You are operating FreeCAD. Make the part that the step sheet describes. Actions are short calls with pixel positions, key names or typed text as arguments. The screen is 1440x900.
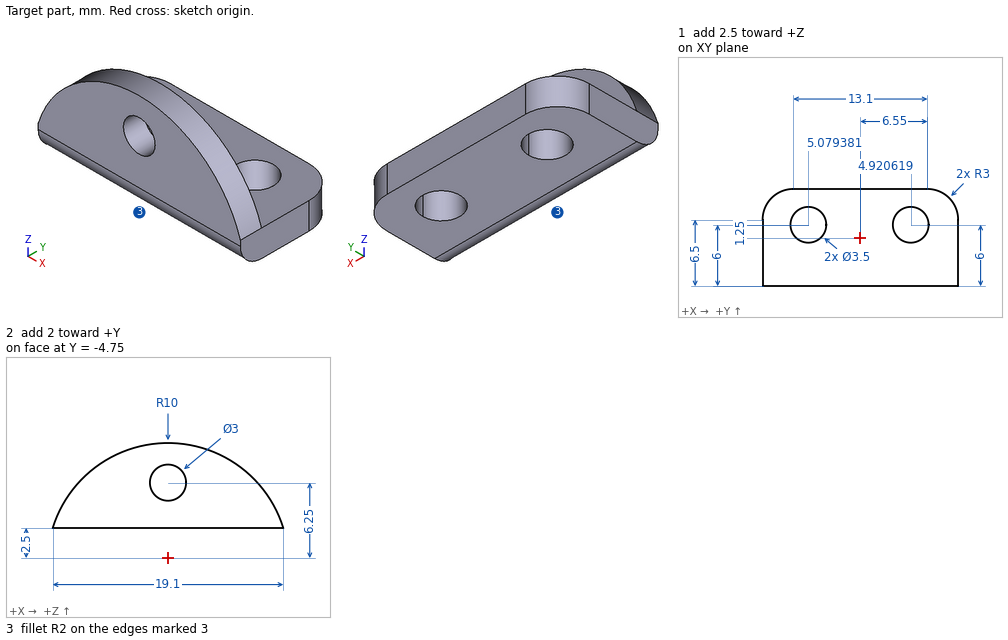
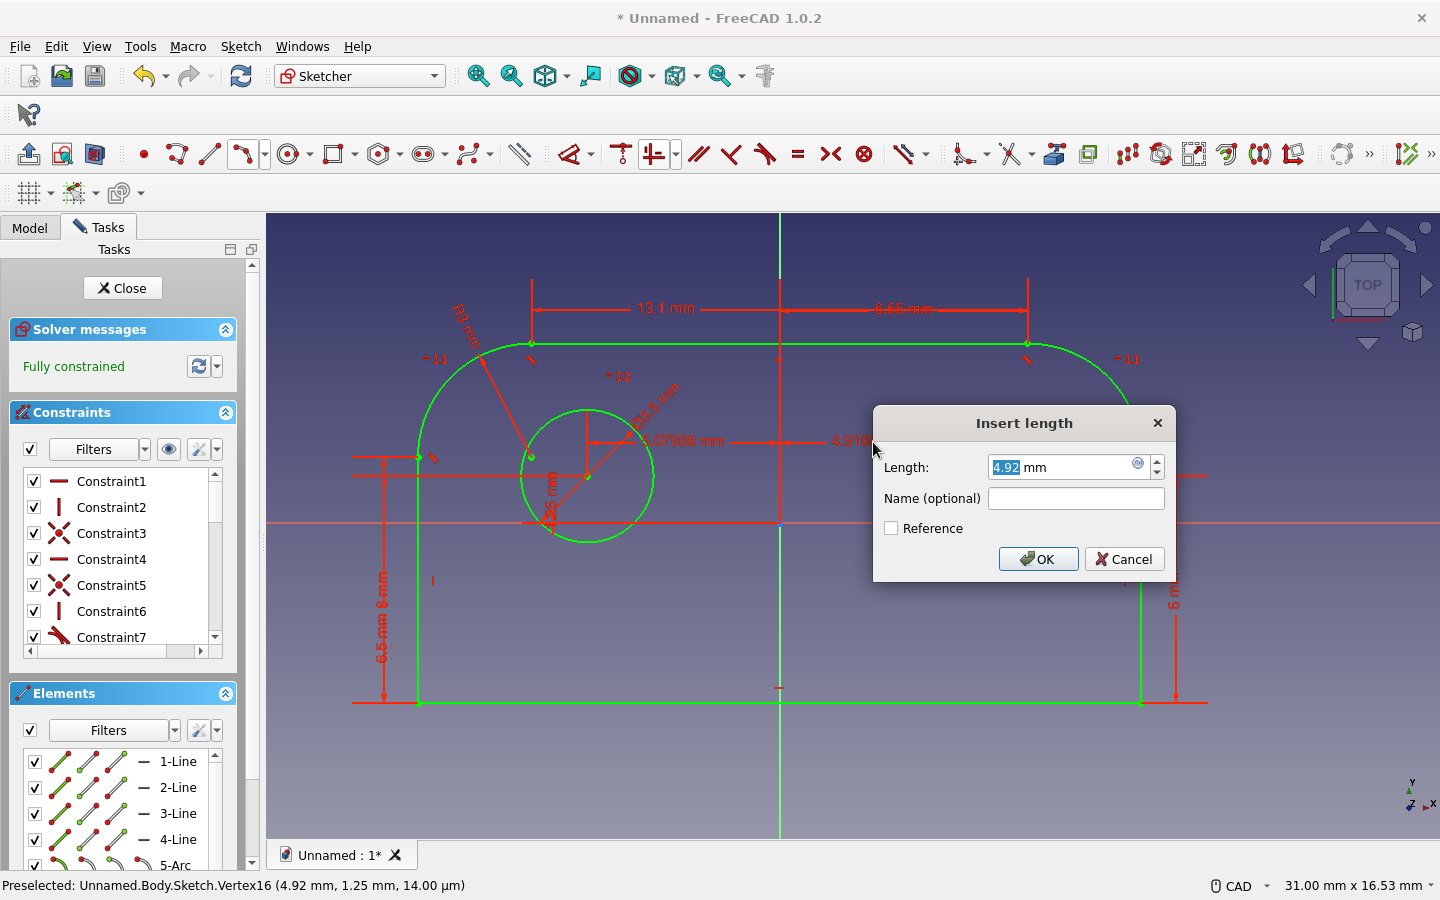
text(4.920619)
key(Return)
key(Escape)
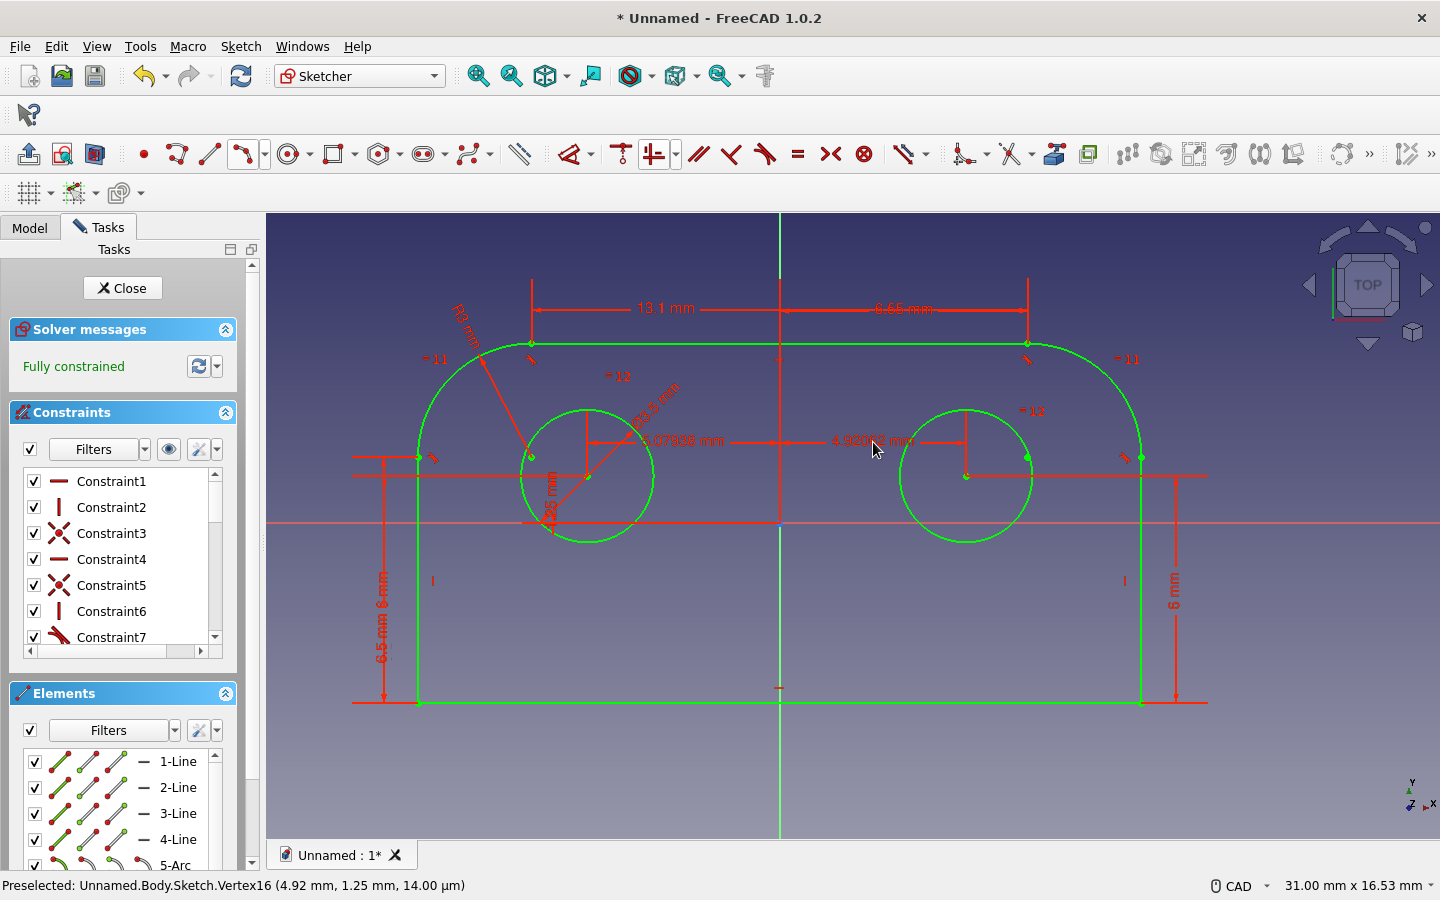
click(123, 288)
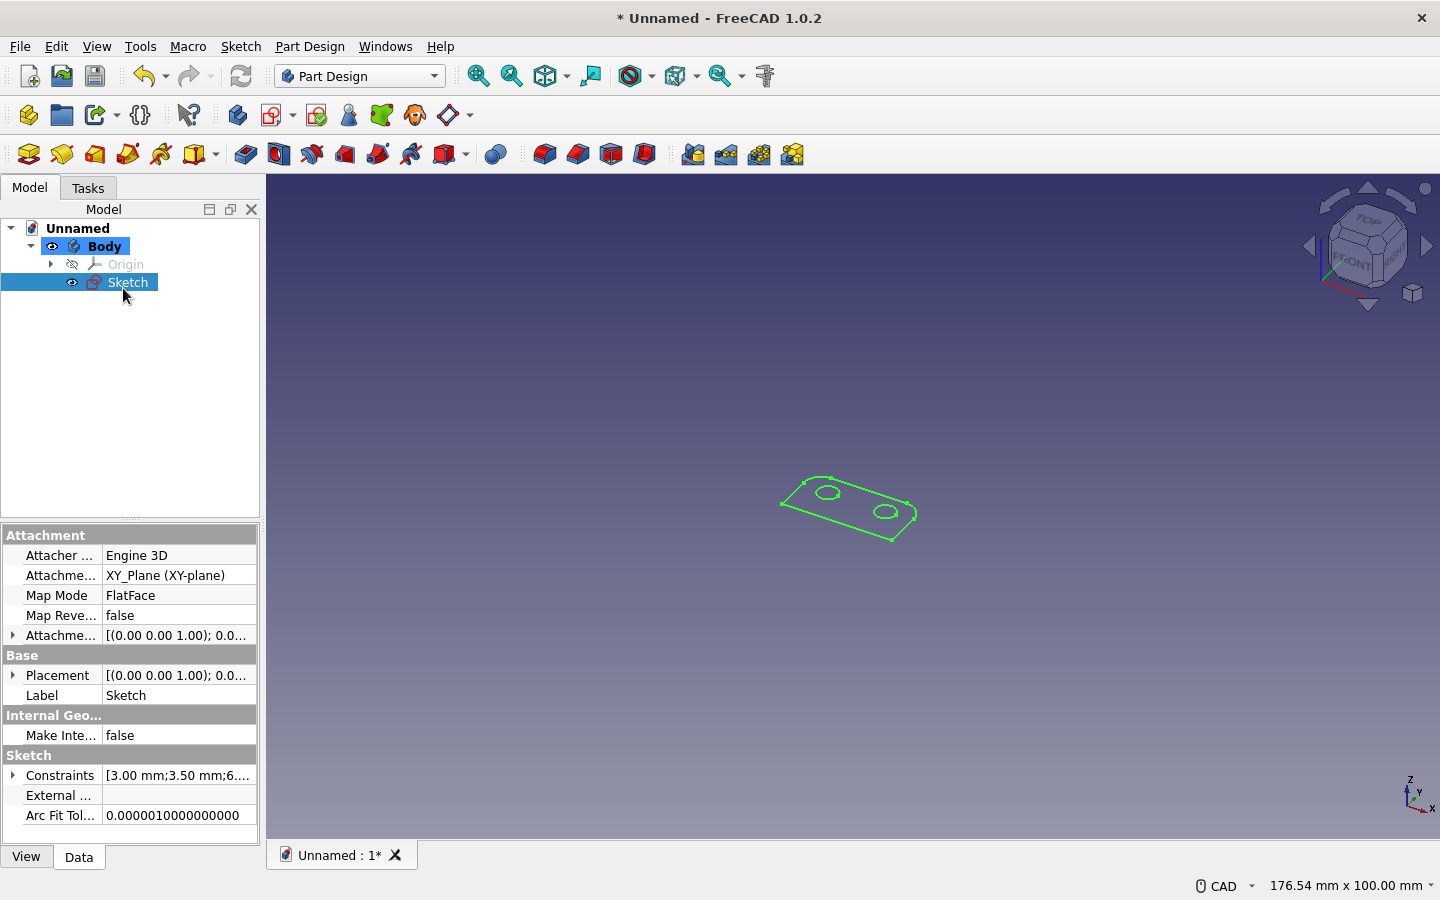
click(29, 154)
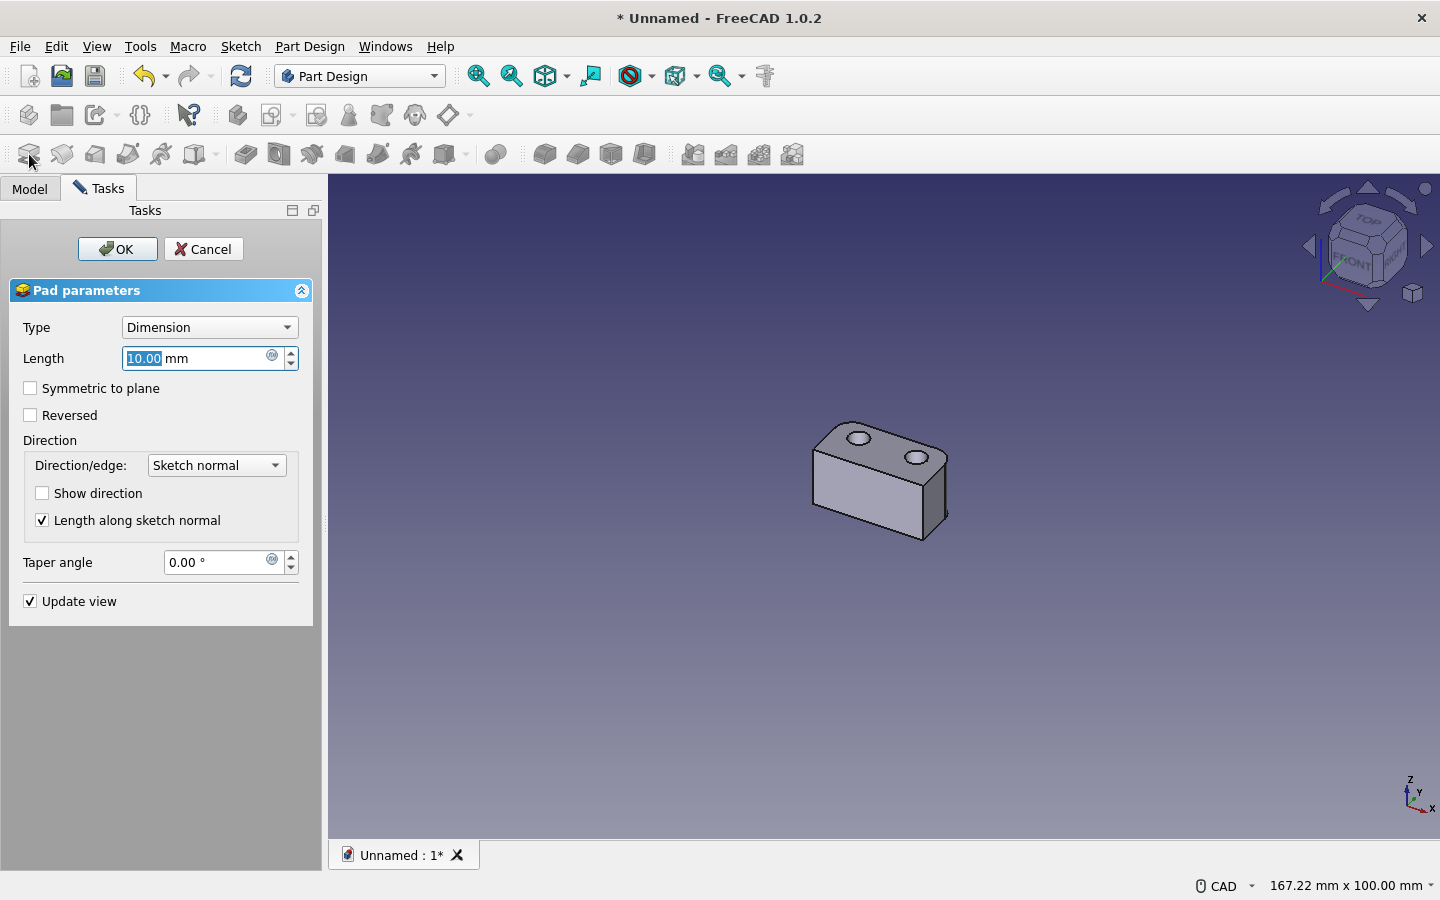
text(2.5)
key(Tab)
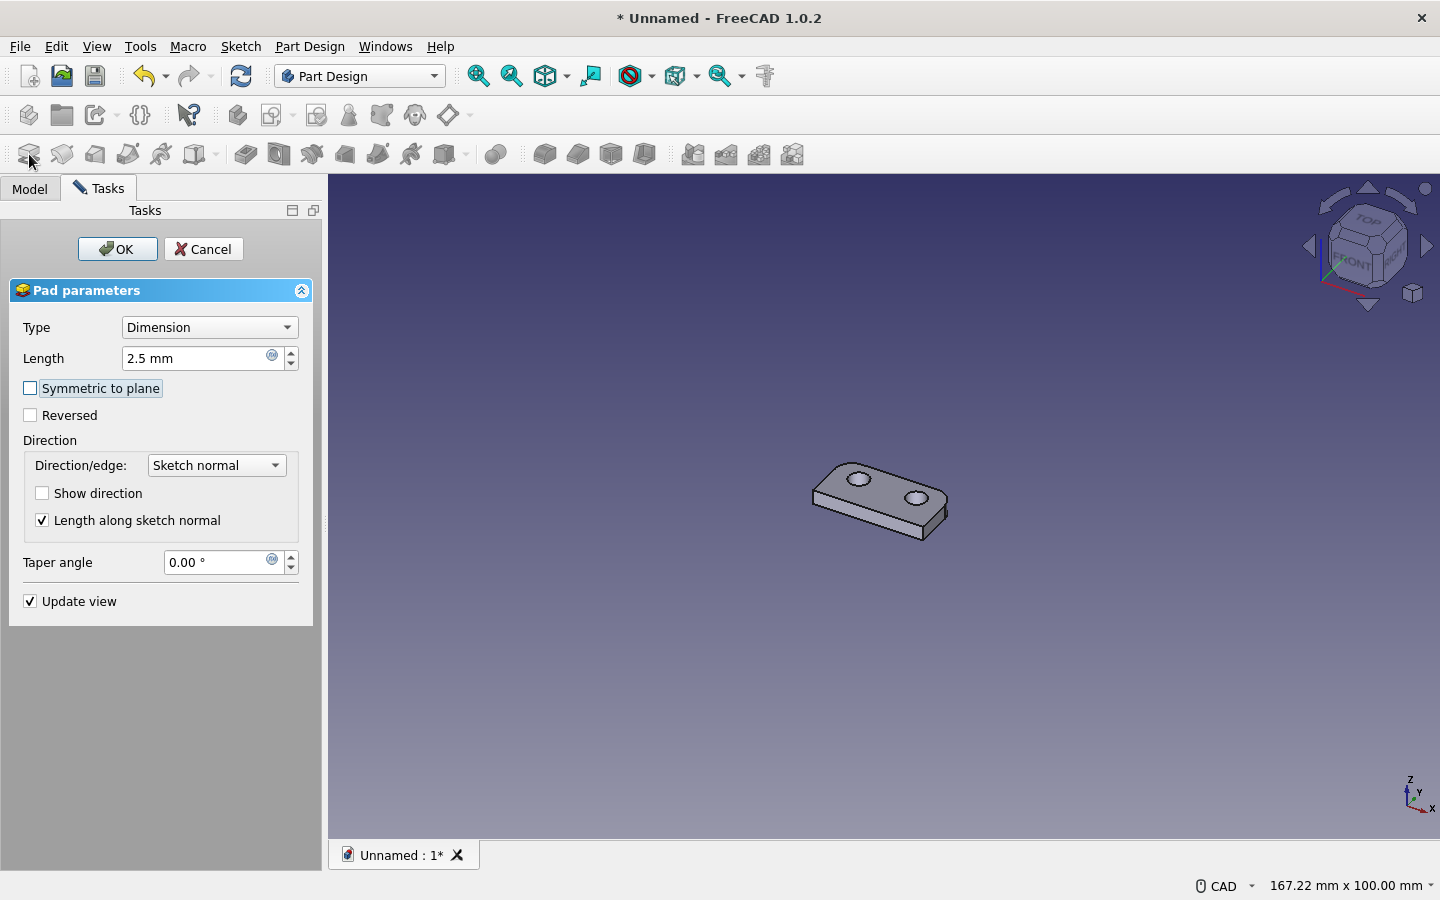
click(118, 249)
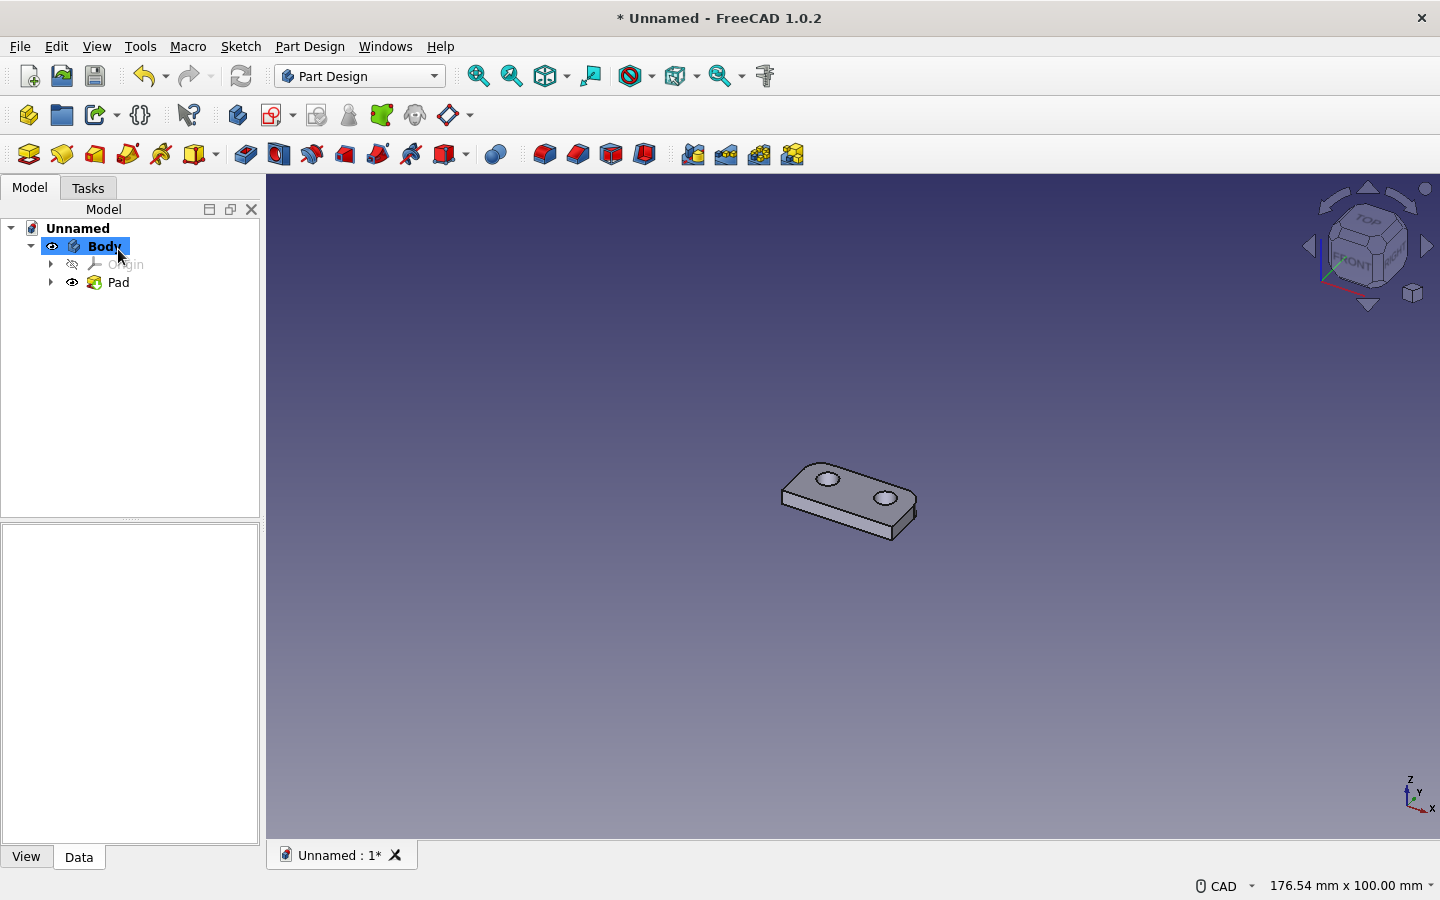
click(479, 76)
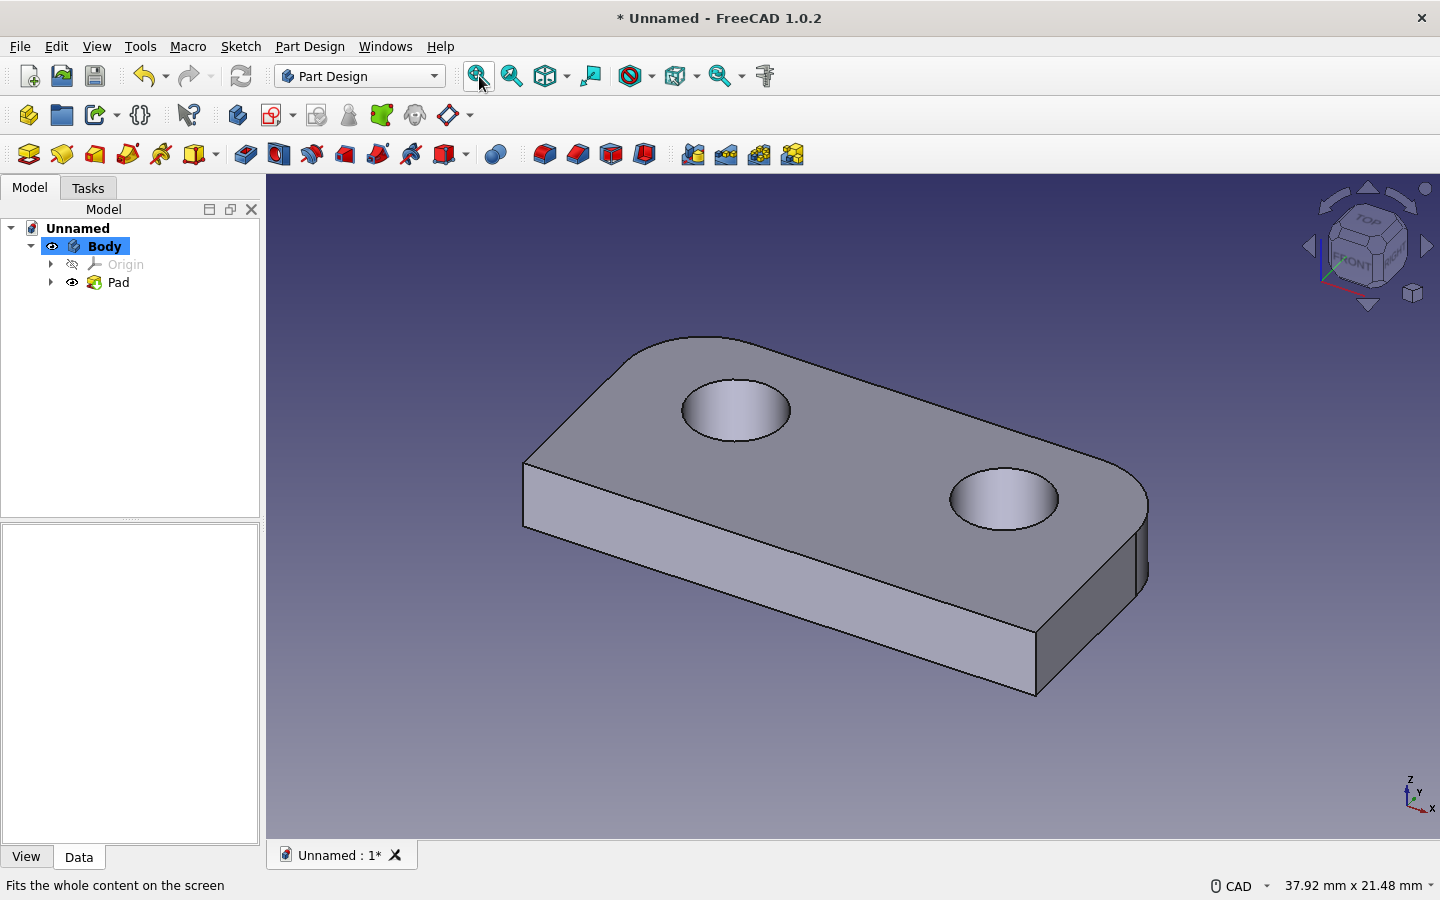
click(999, 651)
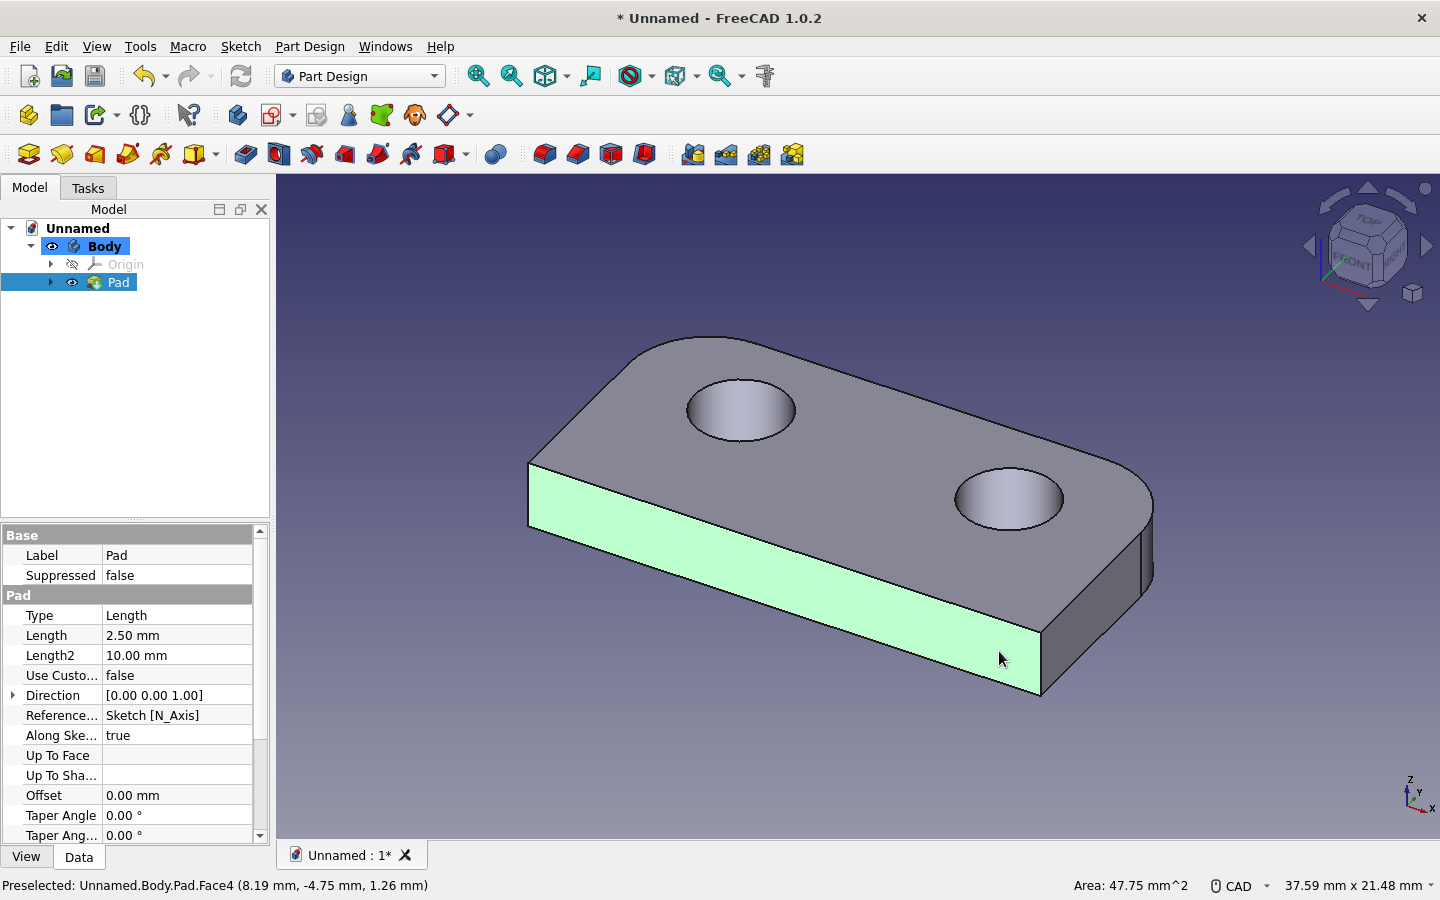
click(270, 116)